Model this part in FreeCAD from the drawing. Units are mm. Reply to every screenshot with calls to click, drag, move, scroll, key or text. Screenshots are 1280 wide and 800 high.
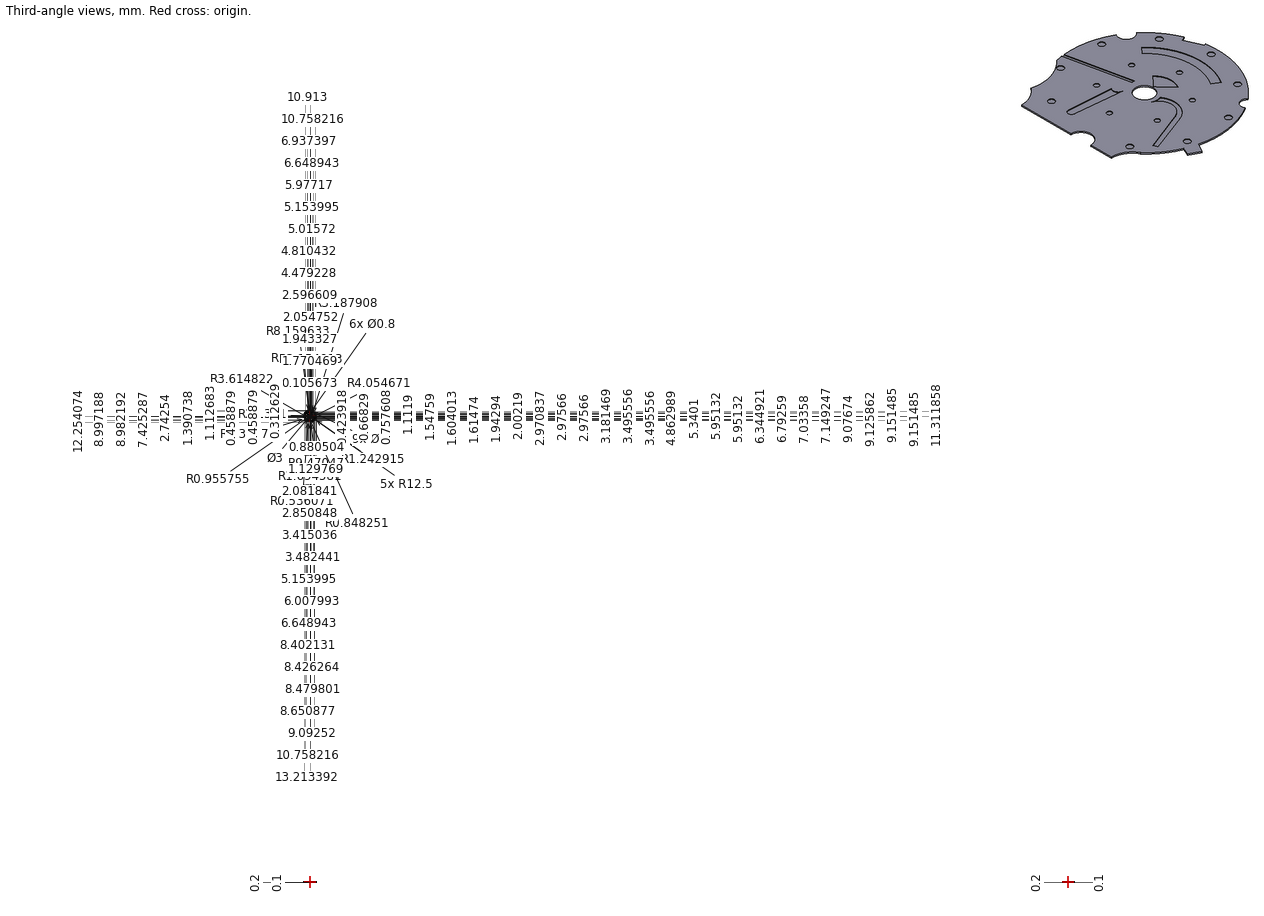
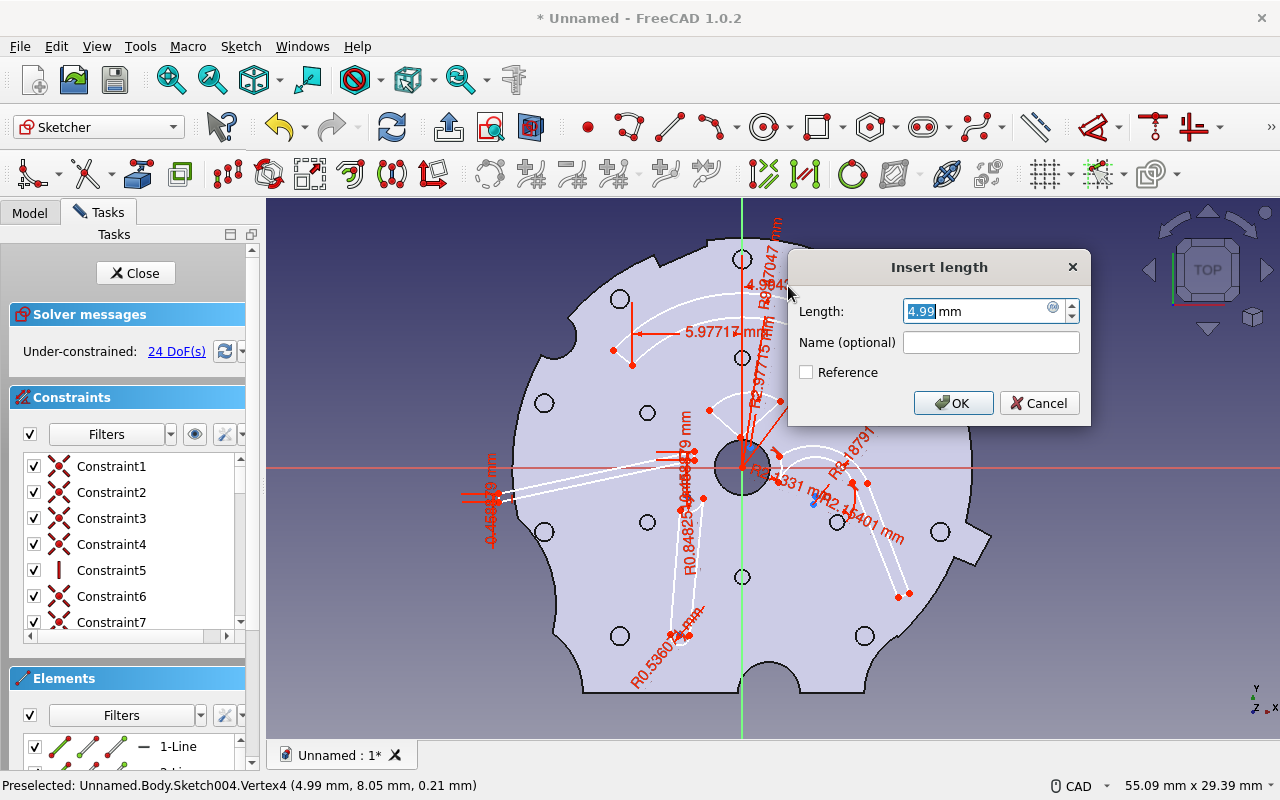
text(5.01572)
key(Return)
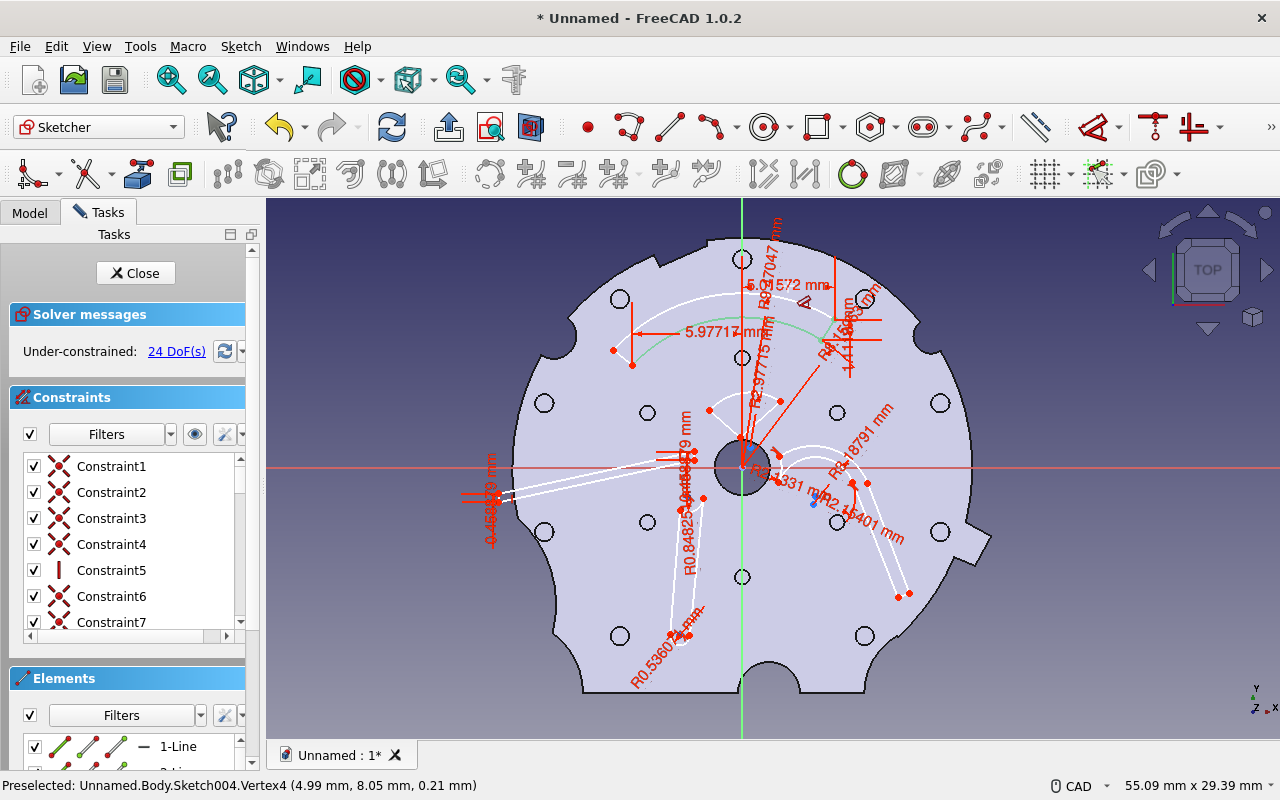
scroll(690, 636, up, 2)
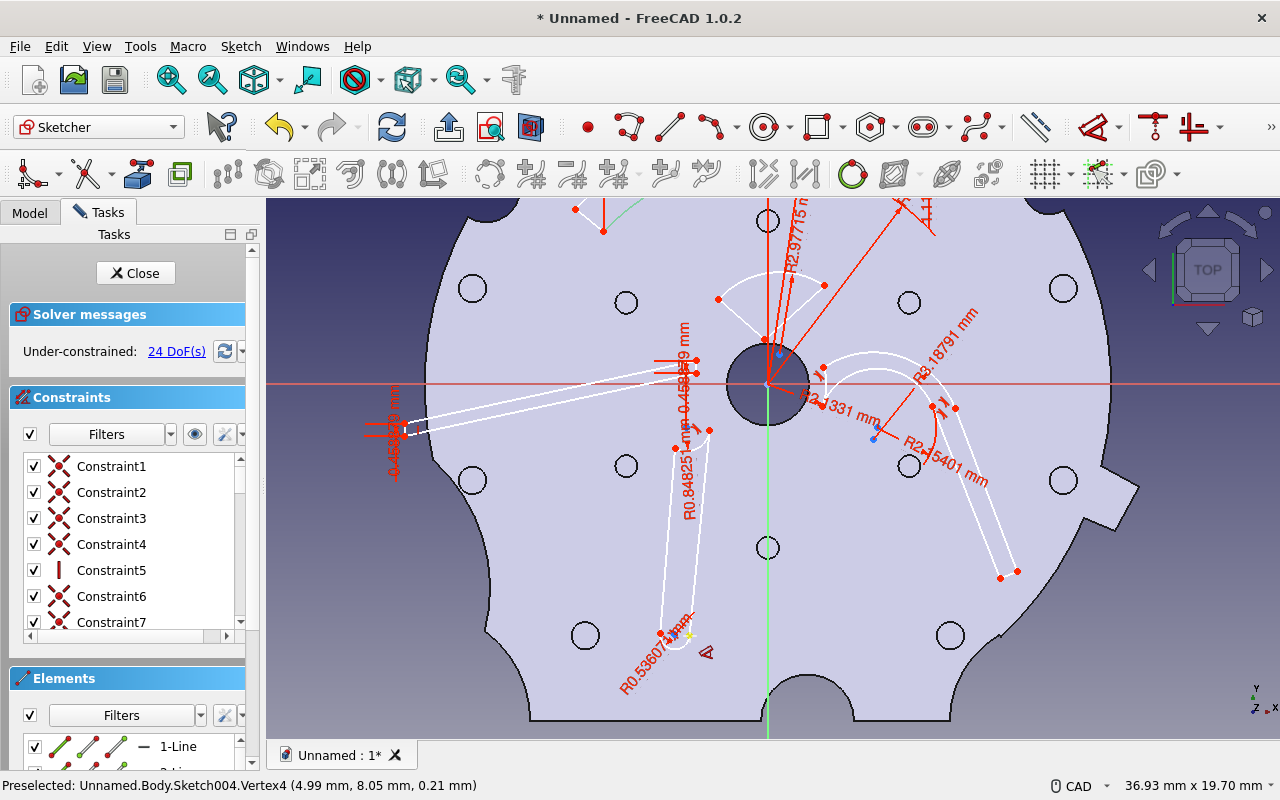
click(690, 635)
click(802, 510)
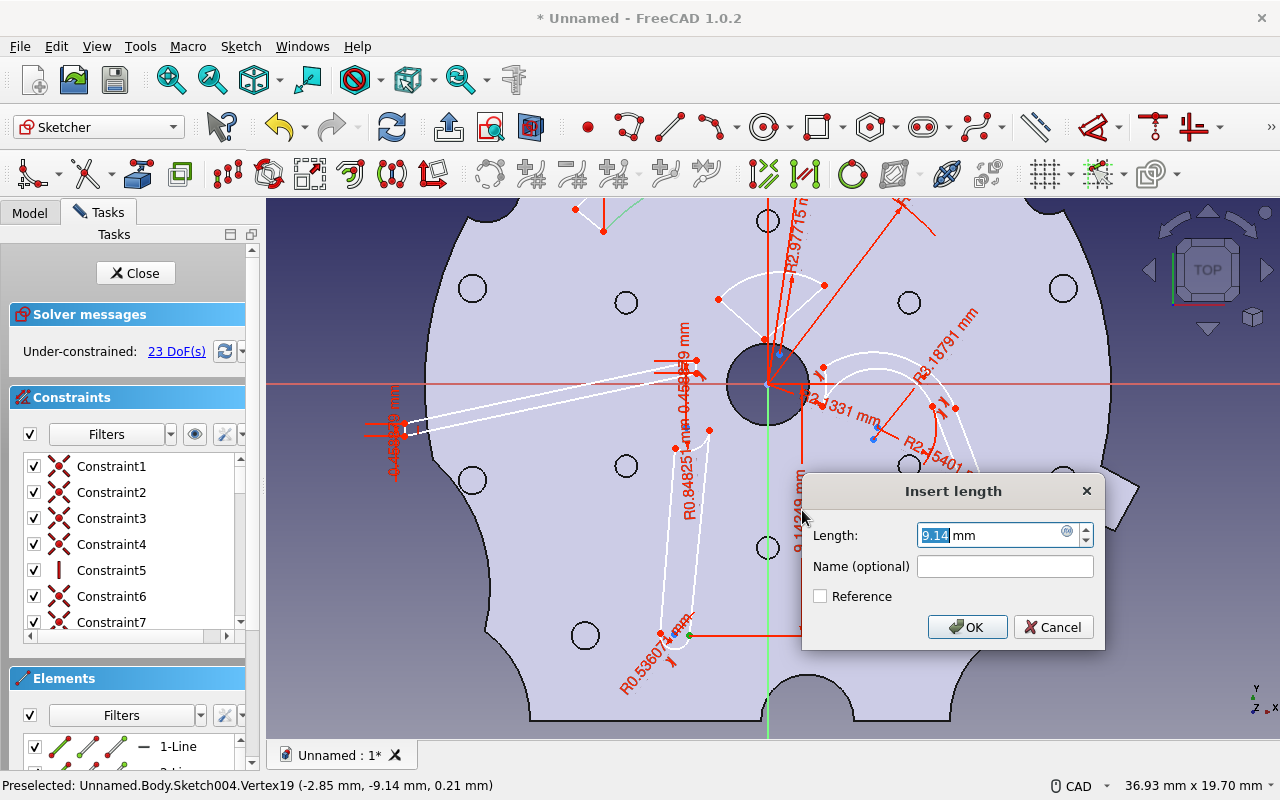
text(9.07674)
key(Return)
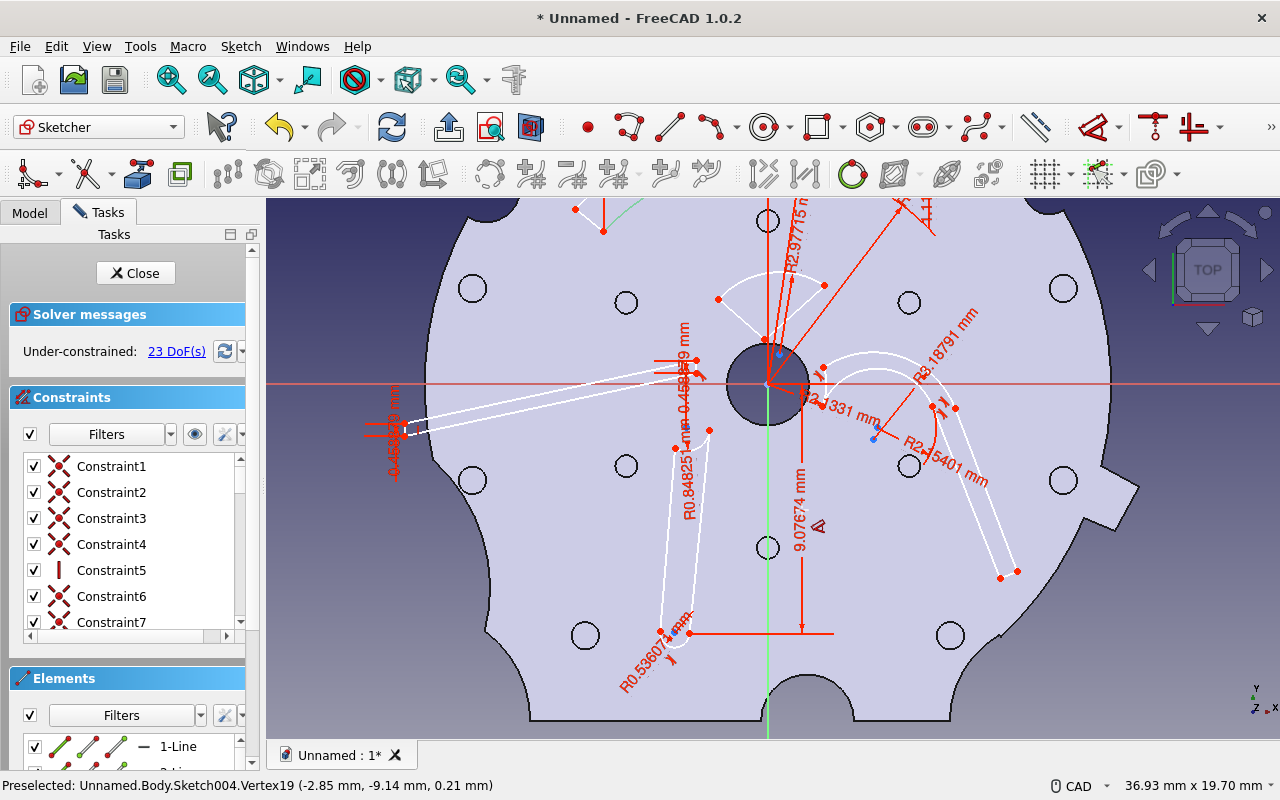
click(1000, 579)
click(1034, 482)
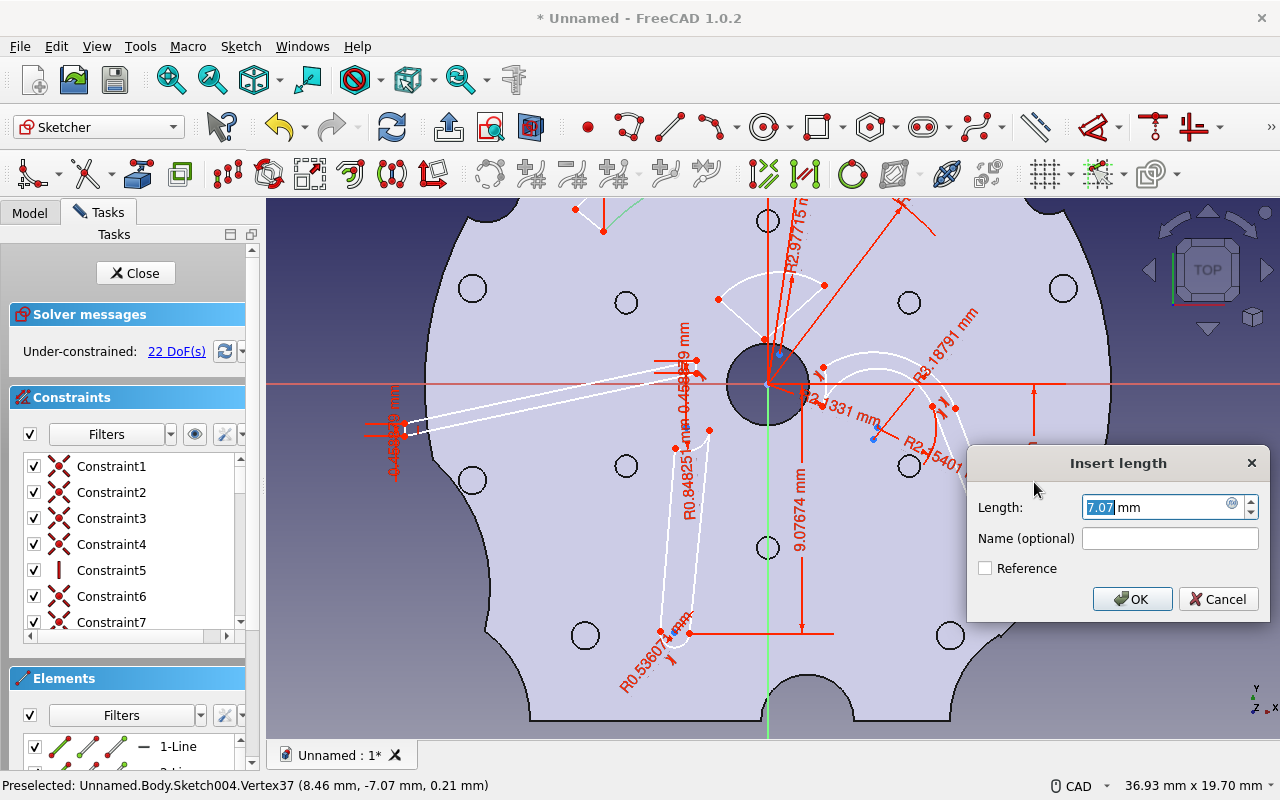
text(7.03358)
key(Return)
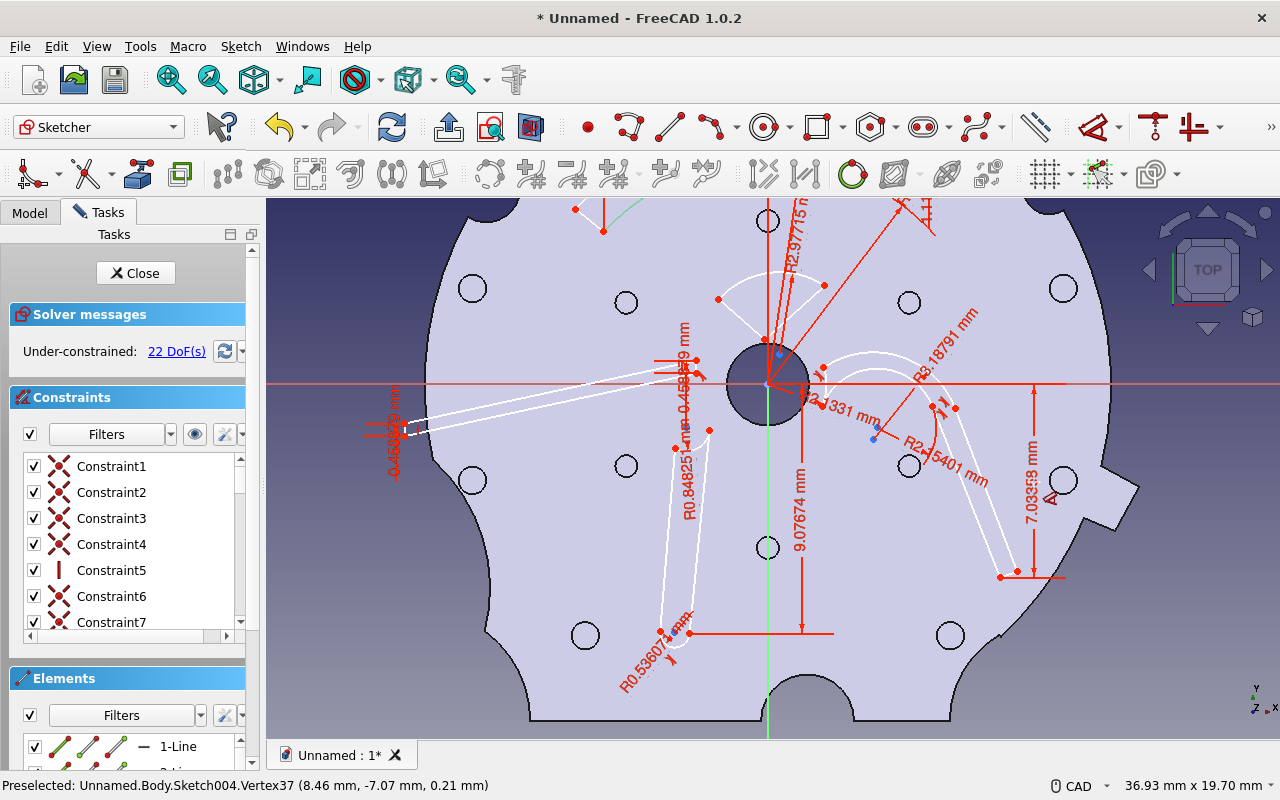
click(1017, 572)
click(893, 606)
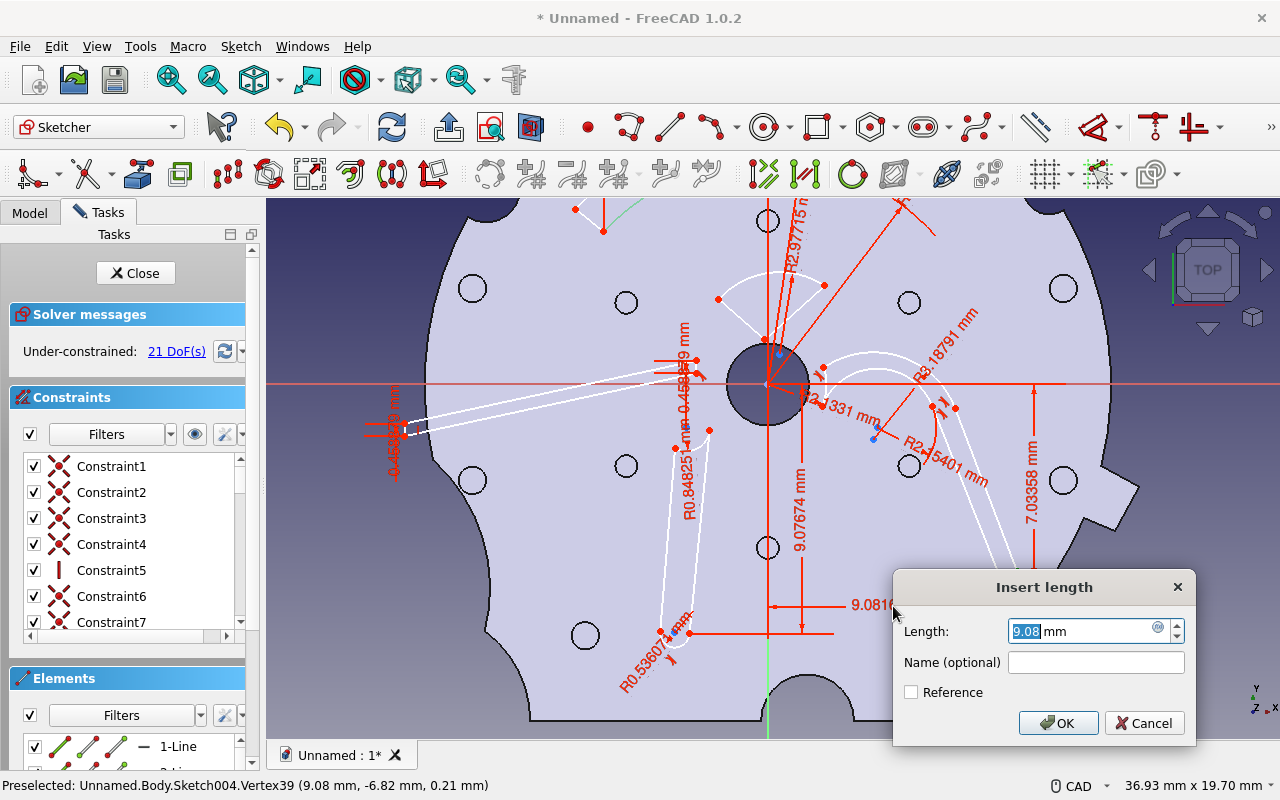
text(9.09252)
key(Return)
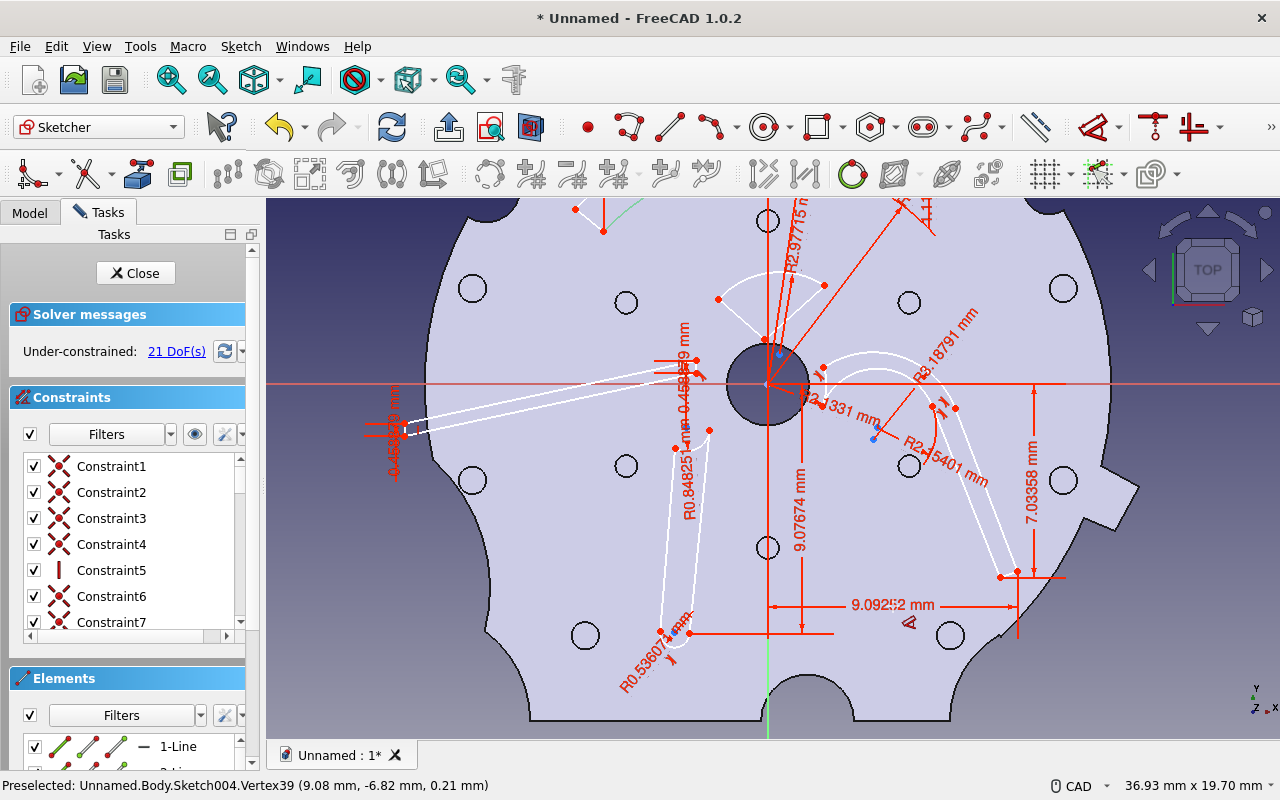
click(1018, 572)
click(1052, 435)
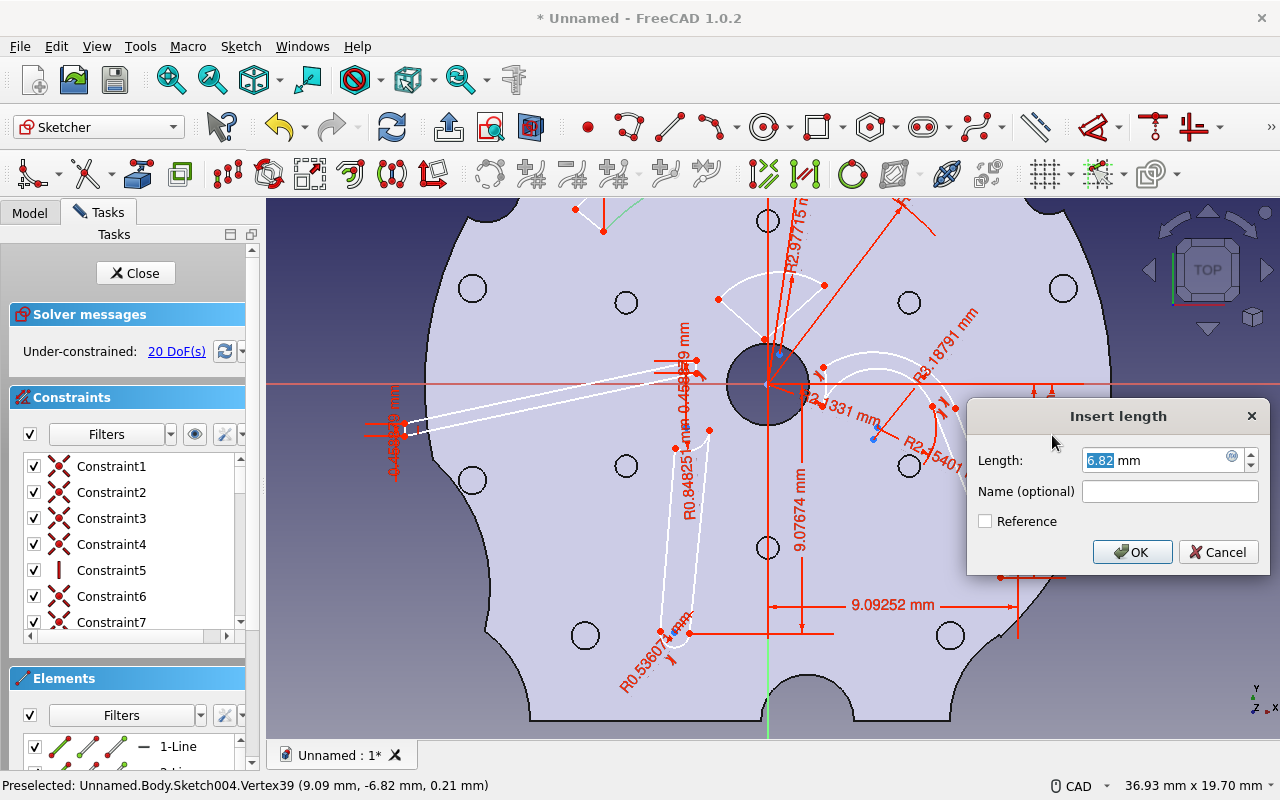
text(6.79259)
key(Return)